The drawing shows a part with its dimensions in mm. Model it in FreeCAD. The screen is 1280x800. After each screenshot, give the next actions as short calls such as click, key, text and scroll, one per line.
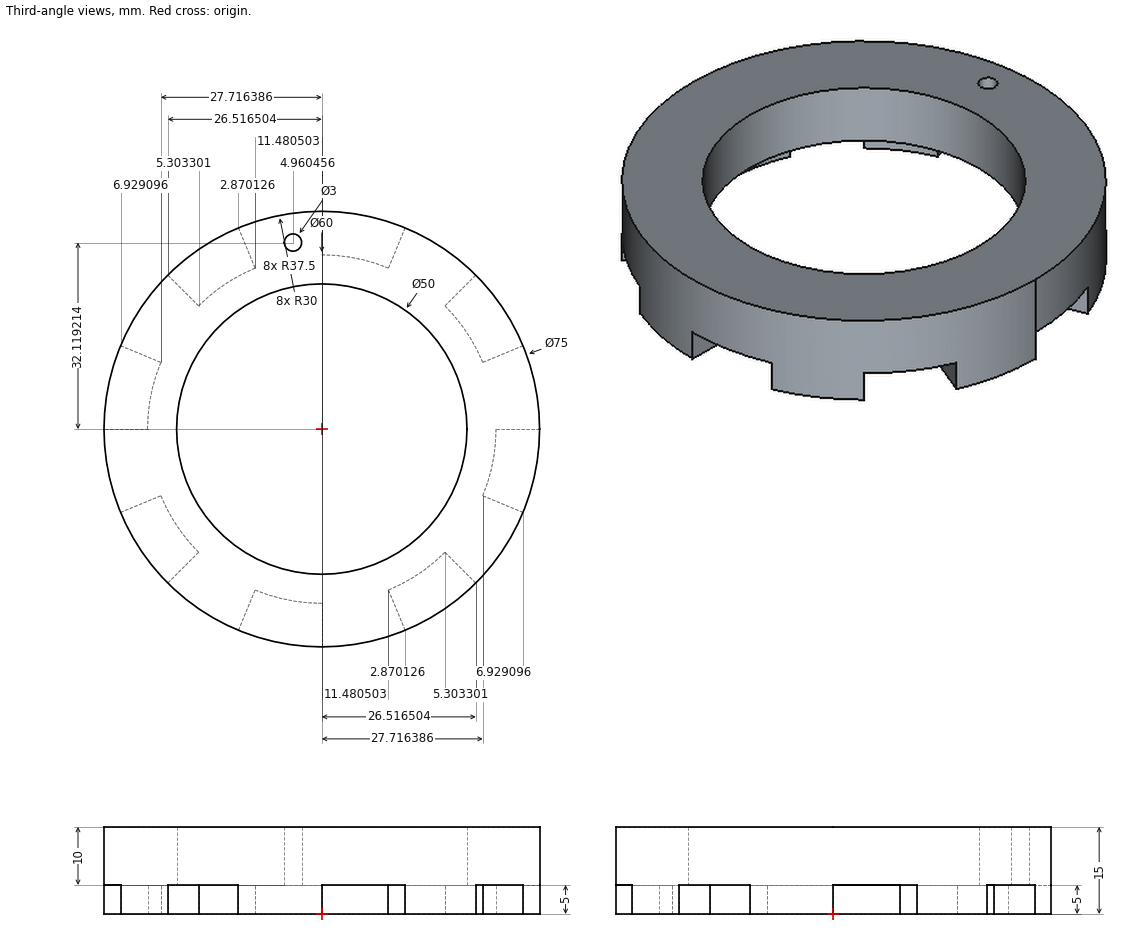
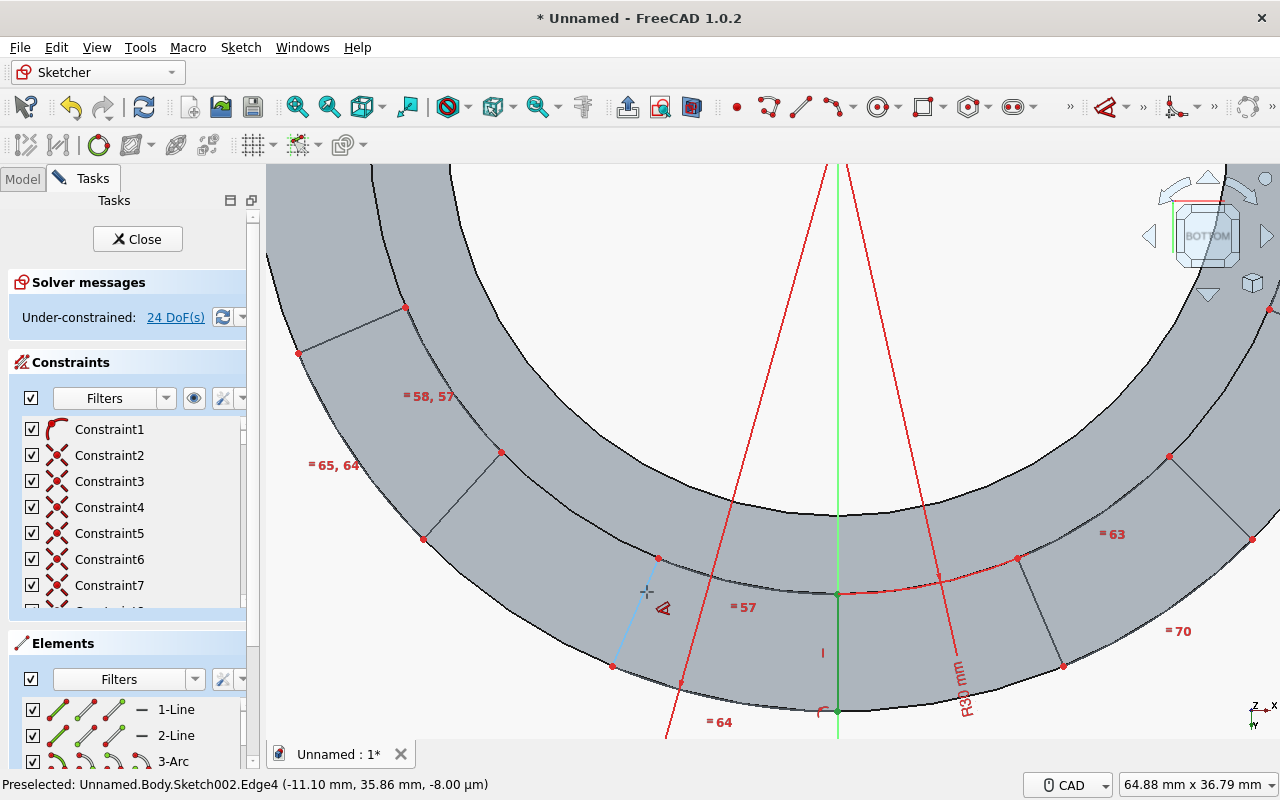
click(645, 591)
click(635, 700)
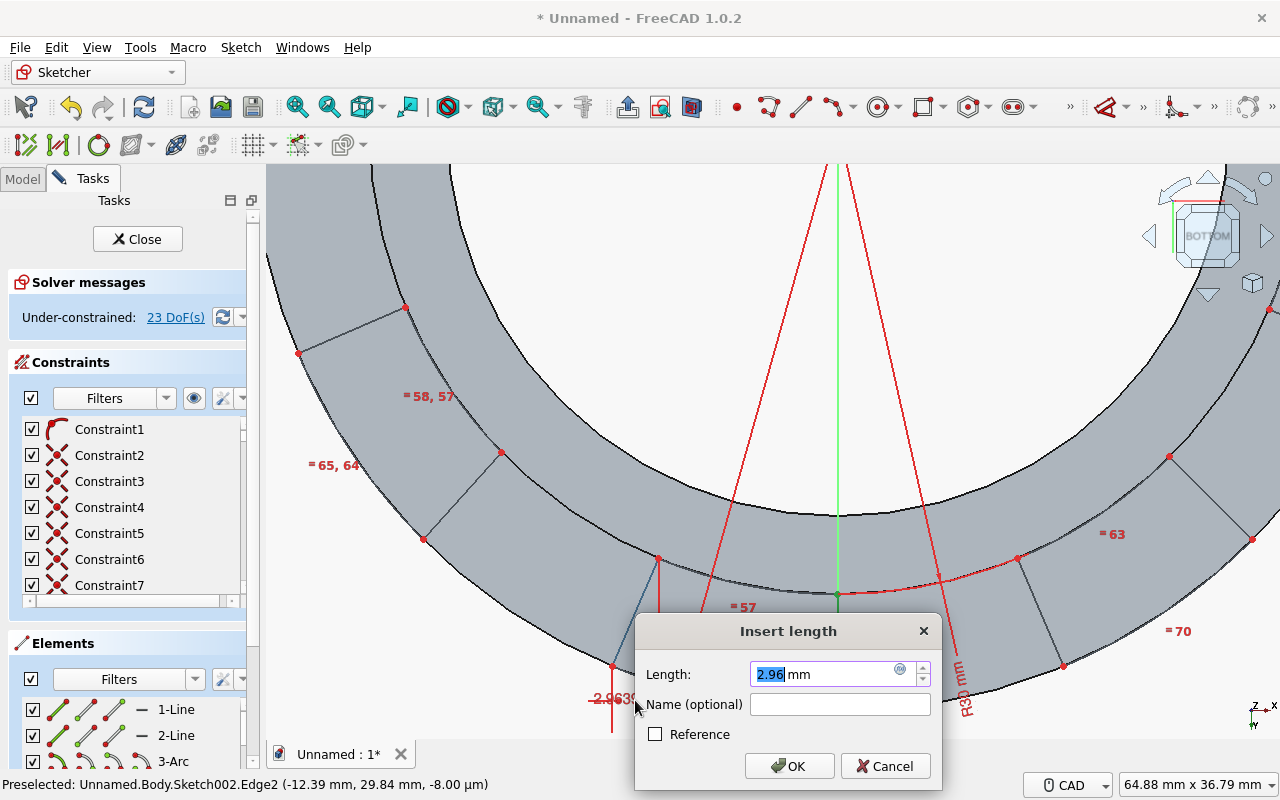
text(2.870126)
key(Return)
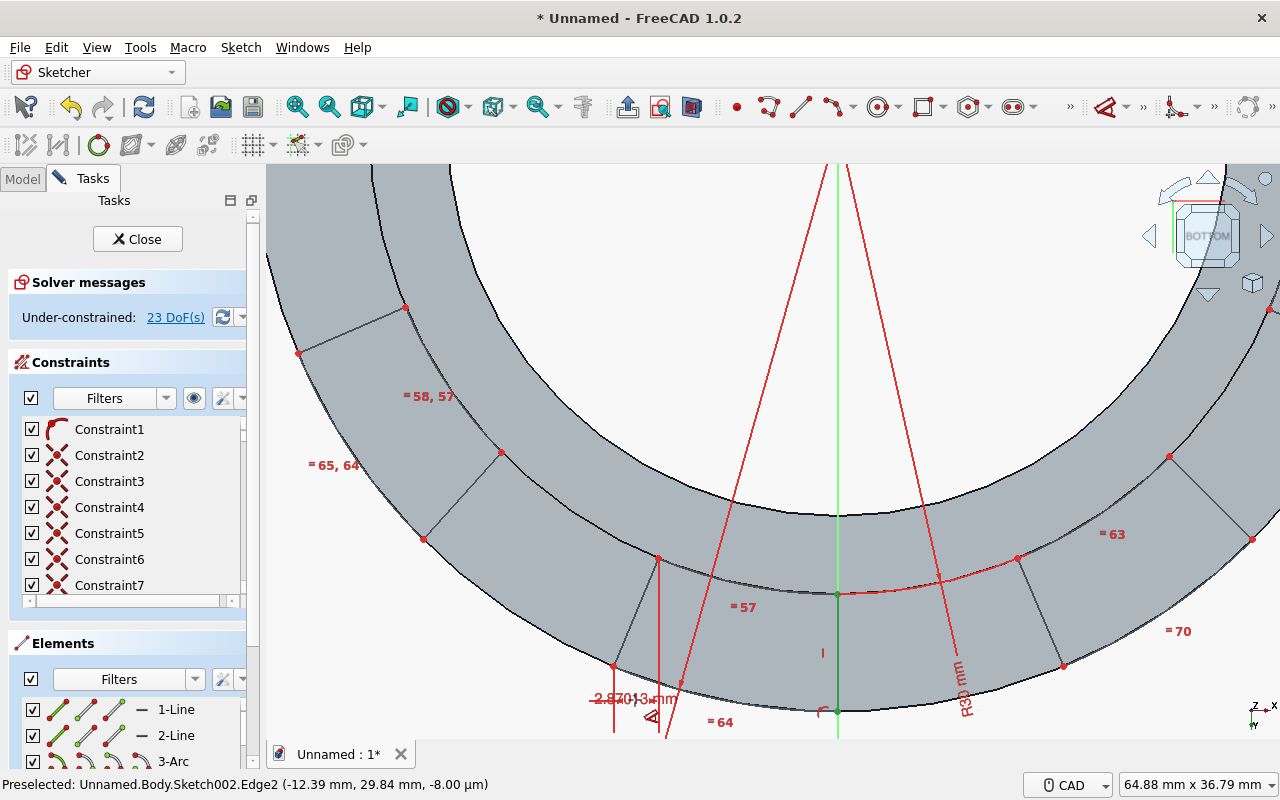
click(447, 513)
click(463, 574)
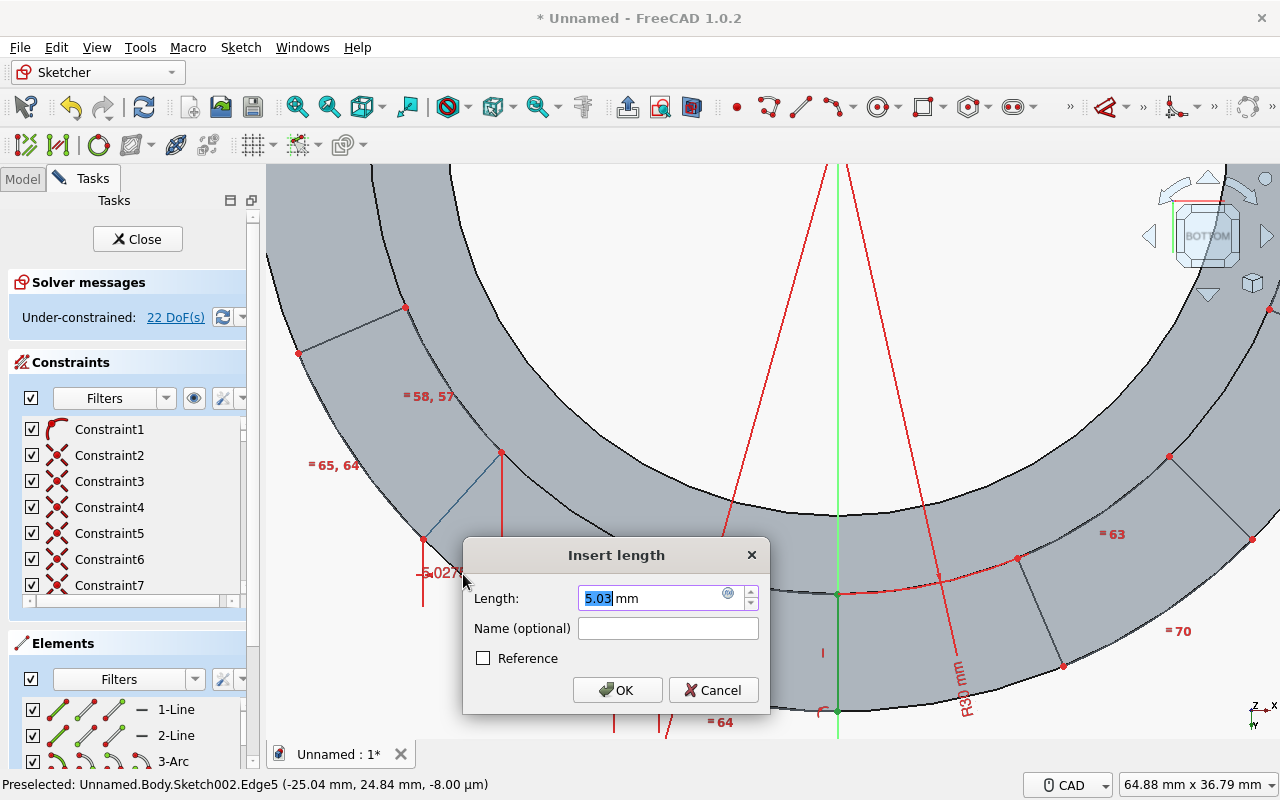
text(5.303301)
key(Return)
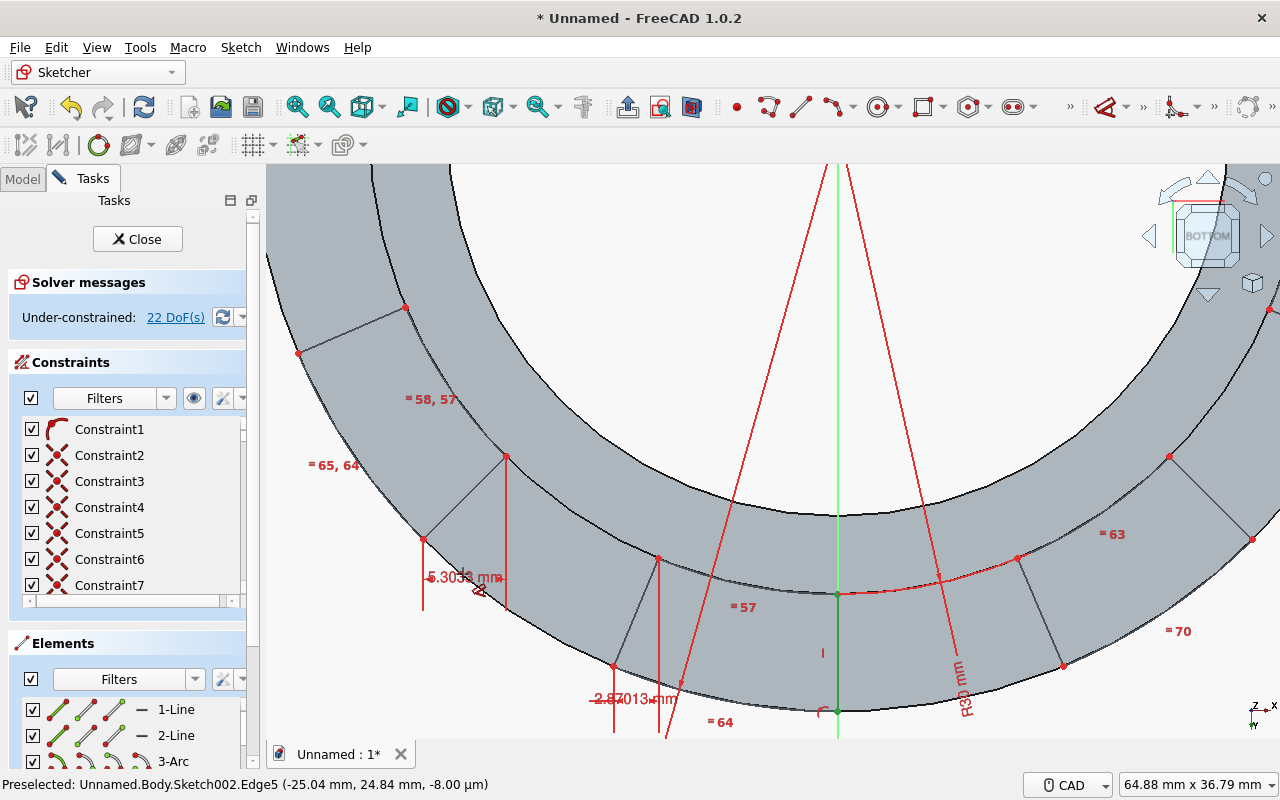
click(373, 321)
click(352, 388)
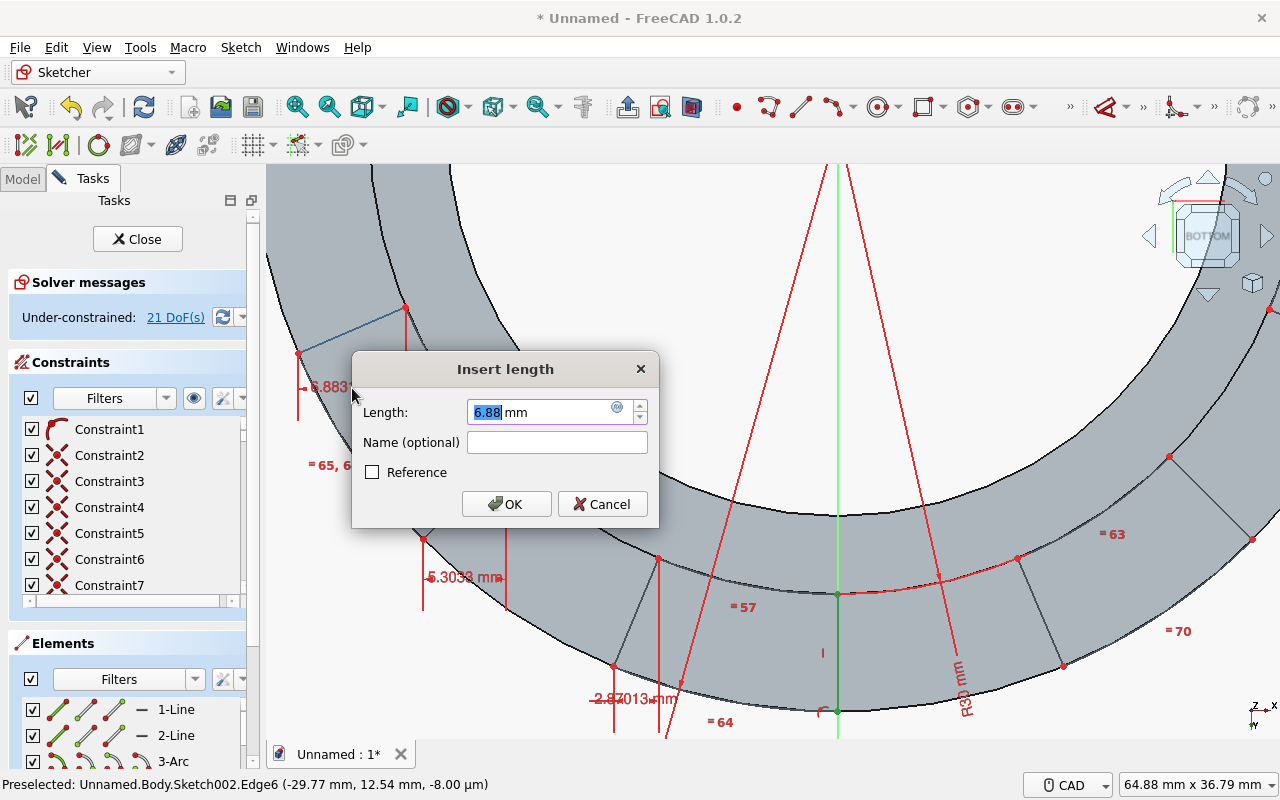
text(6.929096)
key(Return)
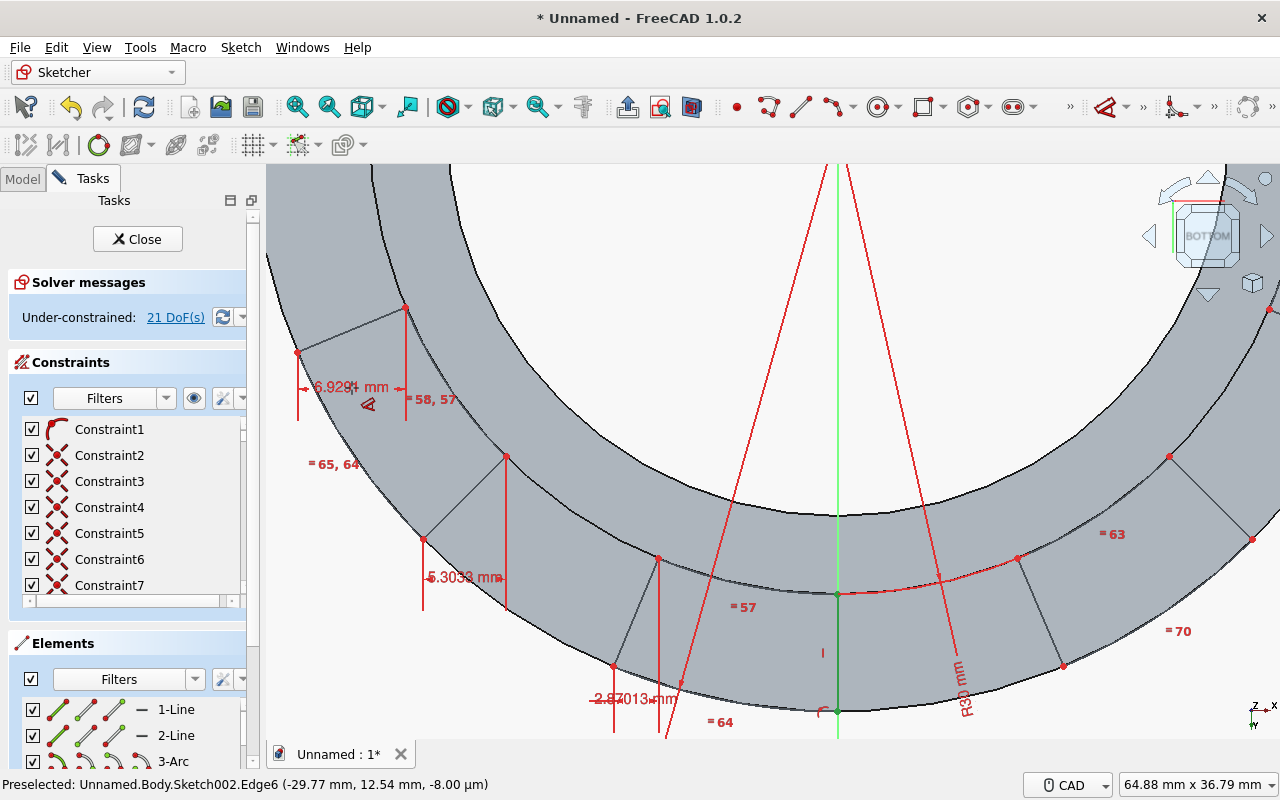
scroll(647, 592, down, 6)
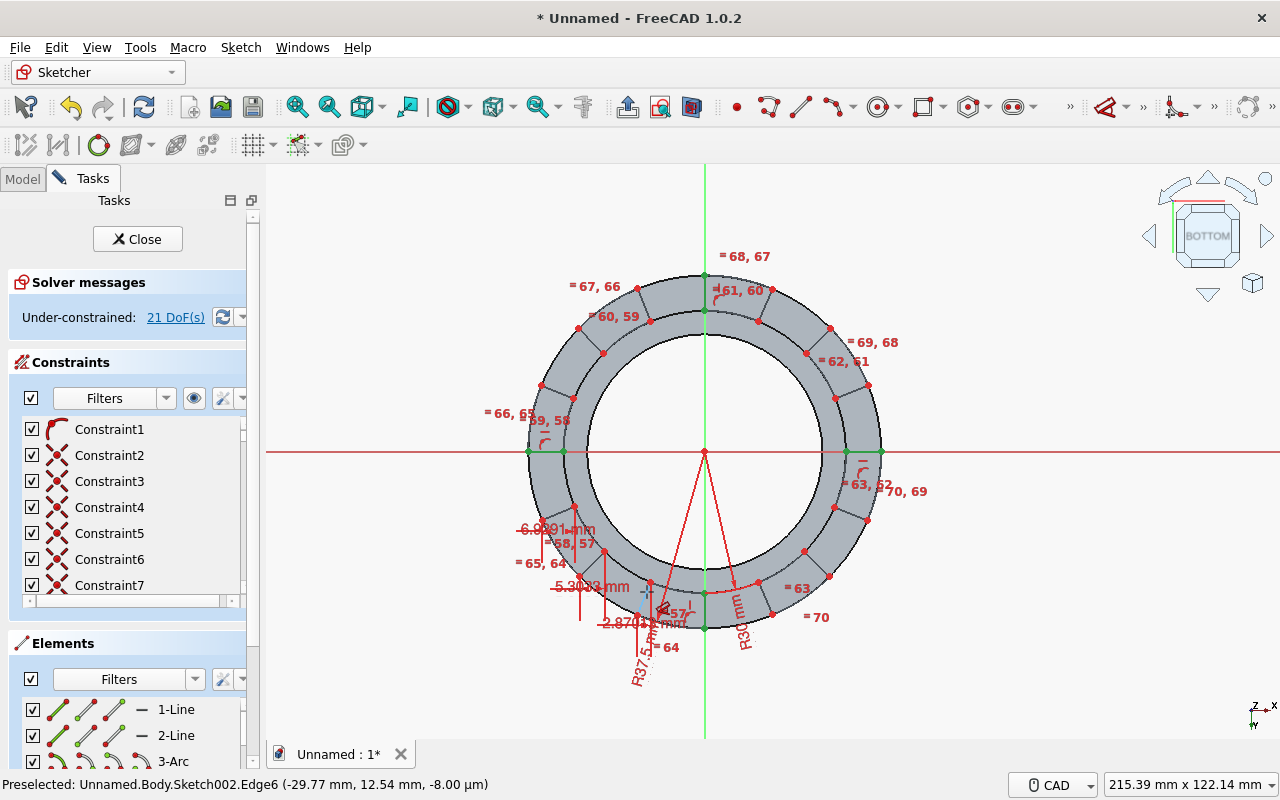
scroll(564, 395, up, 2)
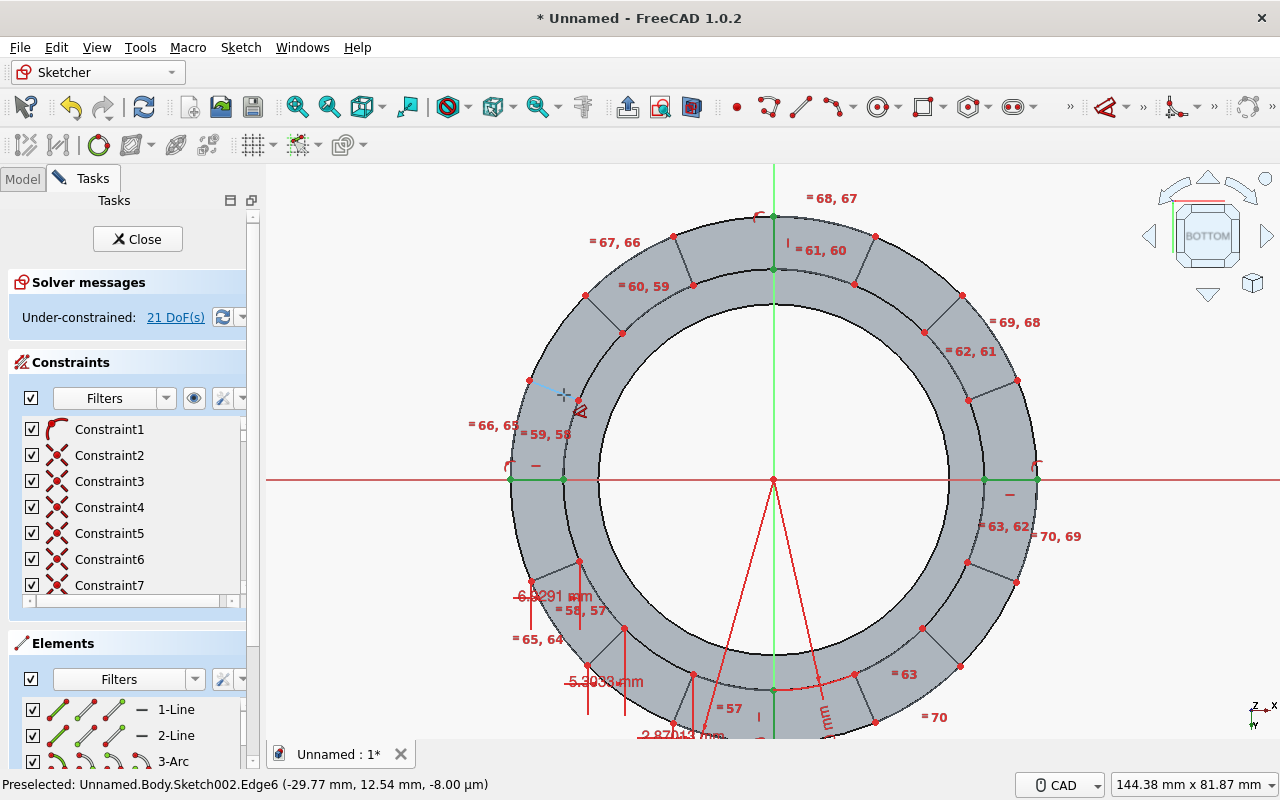
click(564, 395)
click(554, 347)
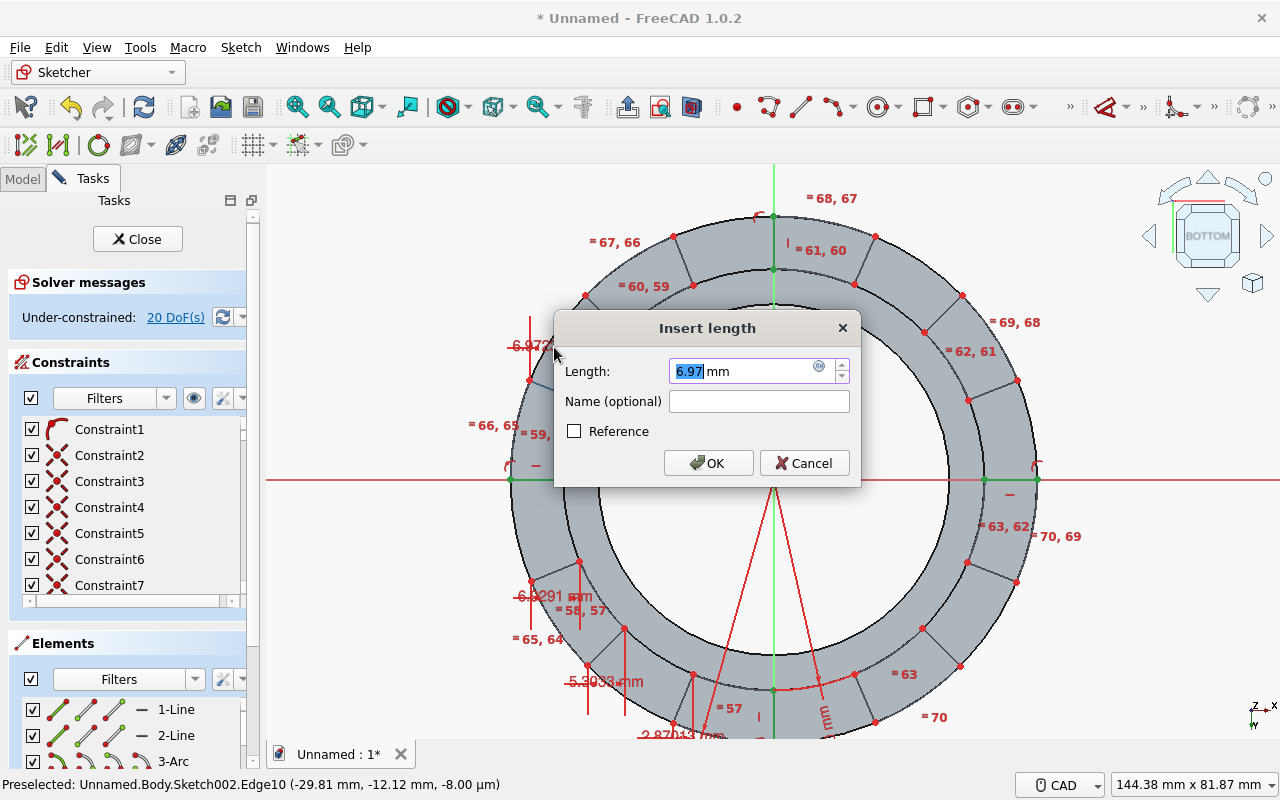
text(6.929096)
key(Return)